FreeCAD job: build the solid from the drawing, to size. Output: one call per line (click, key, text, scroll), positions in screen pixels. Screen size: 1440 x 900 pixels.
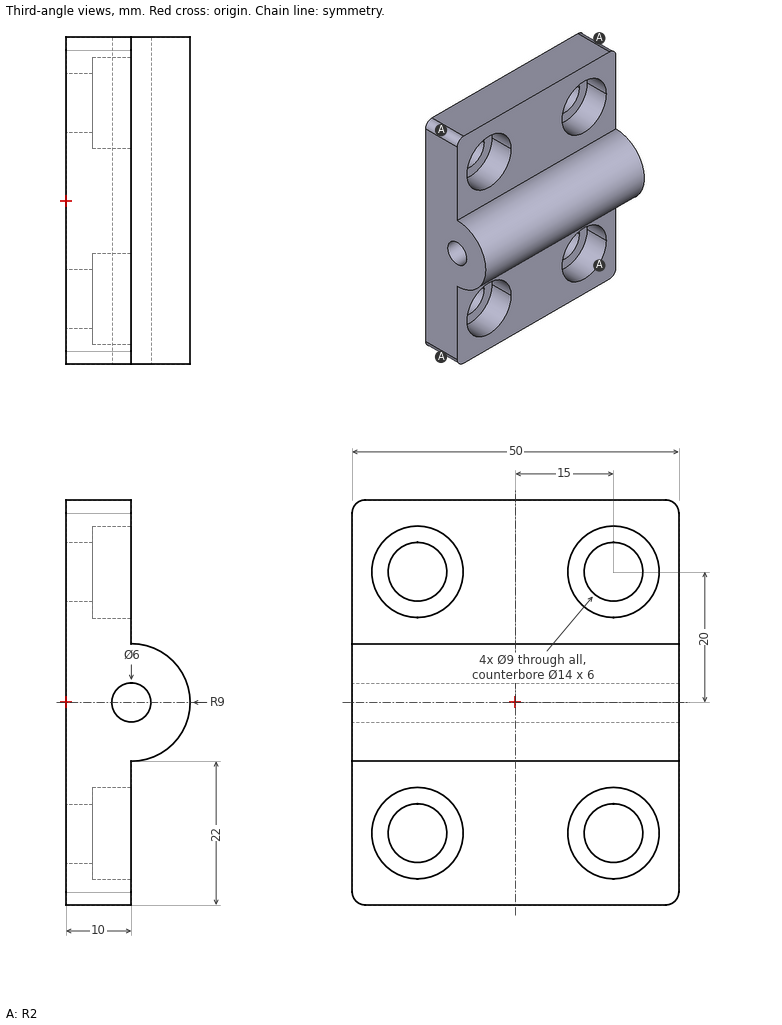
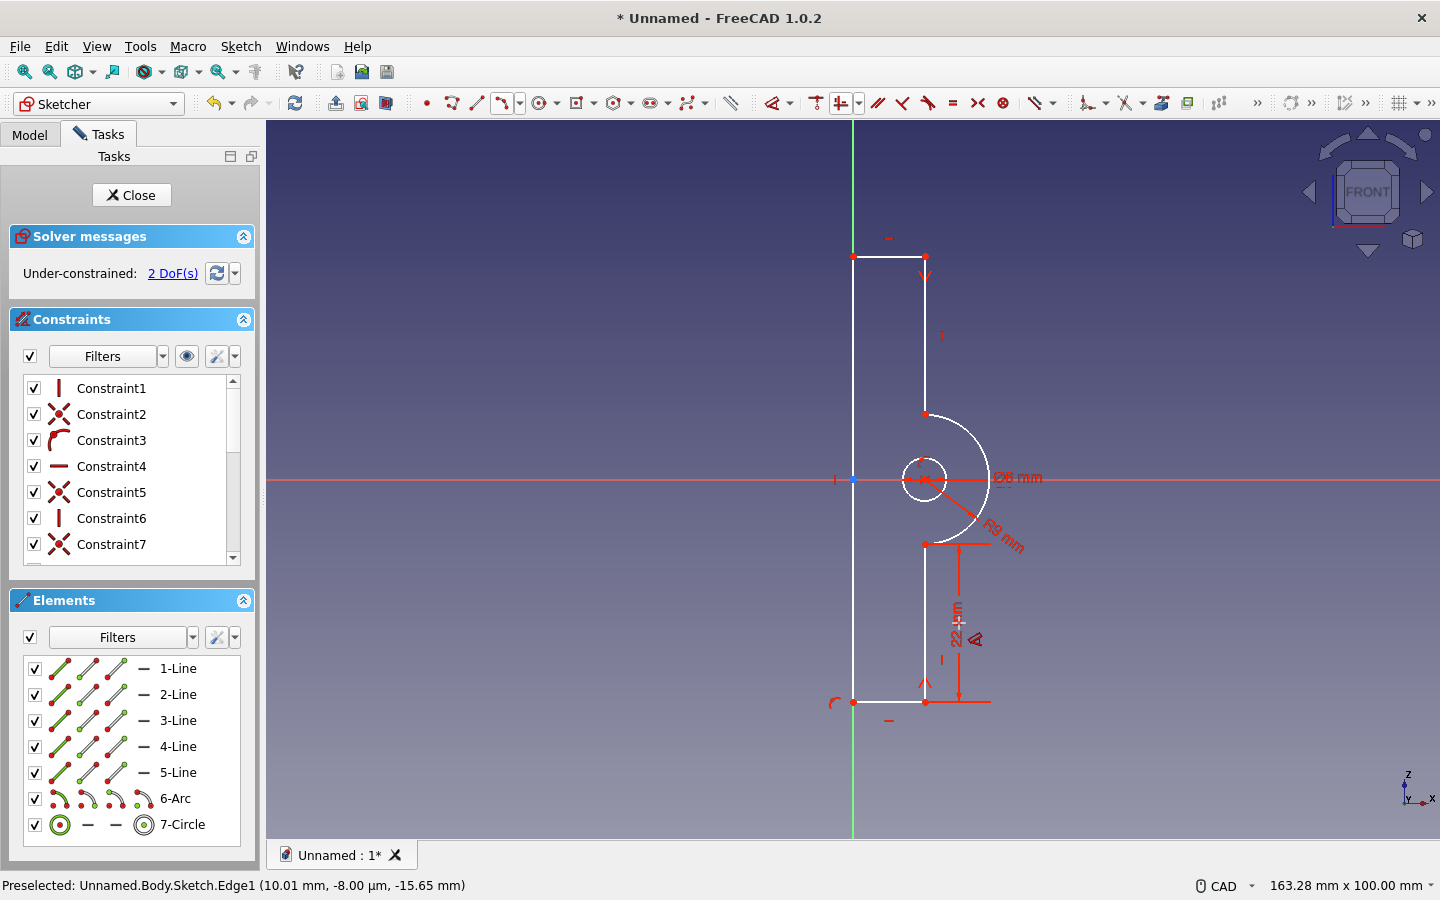
click(903, 702)
click(889, 736)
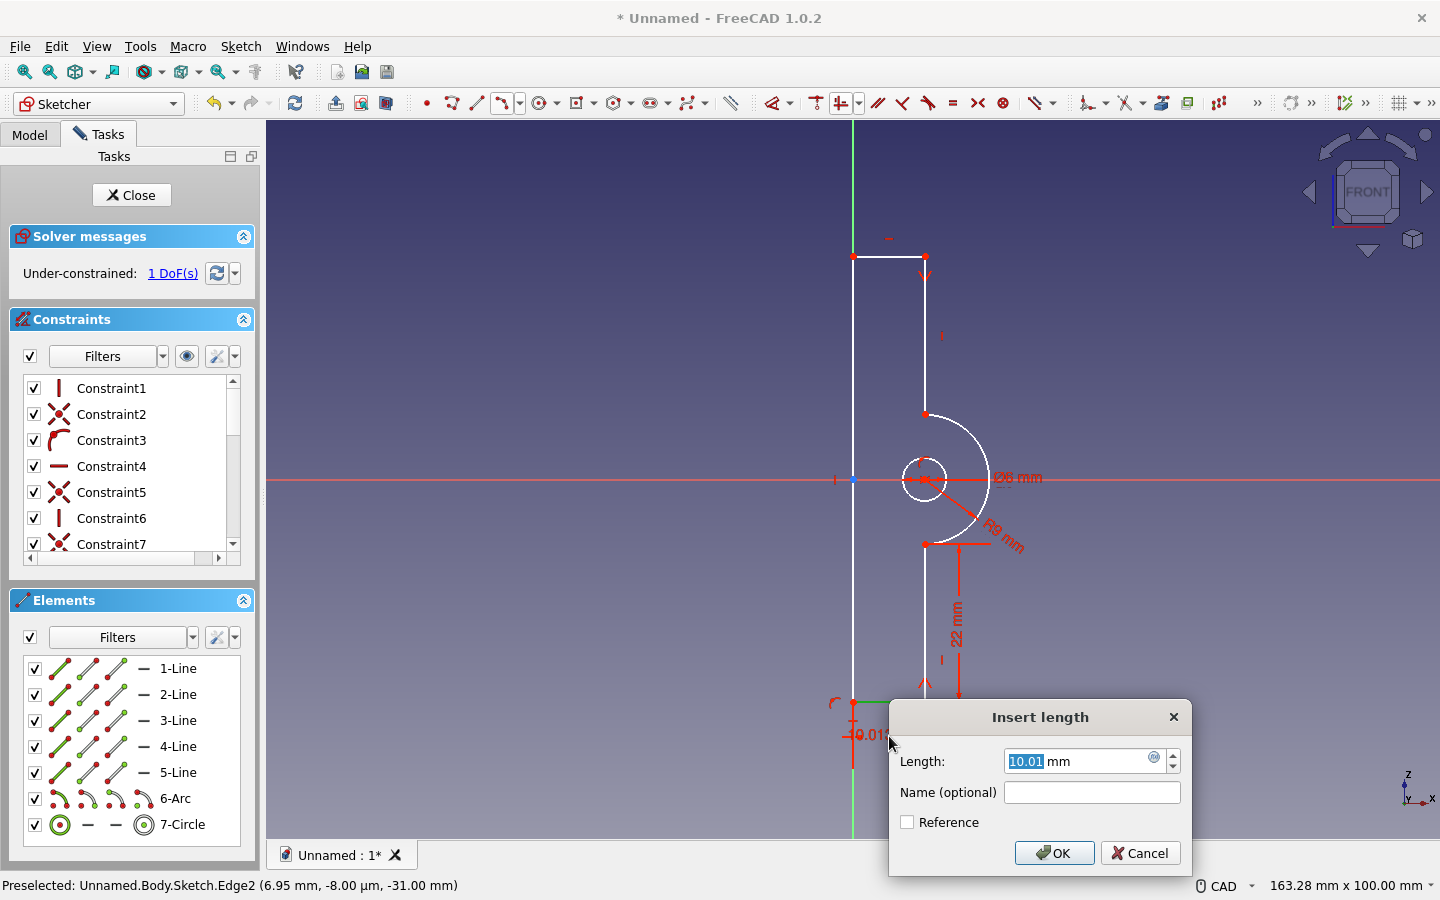
text(10)
key(Return)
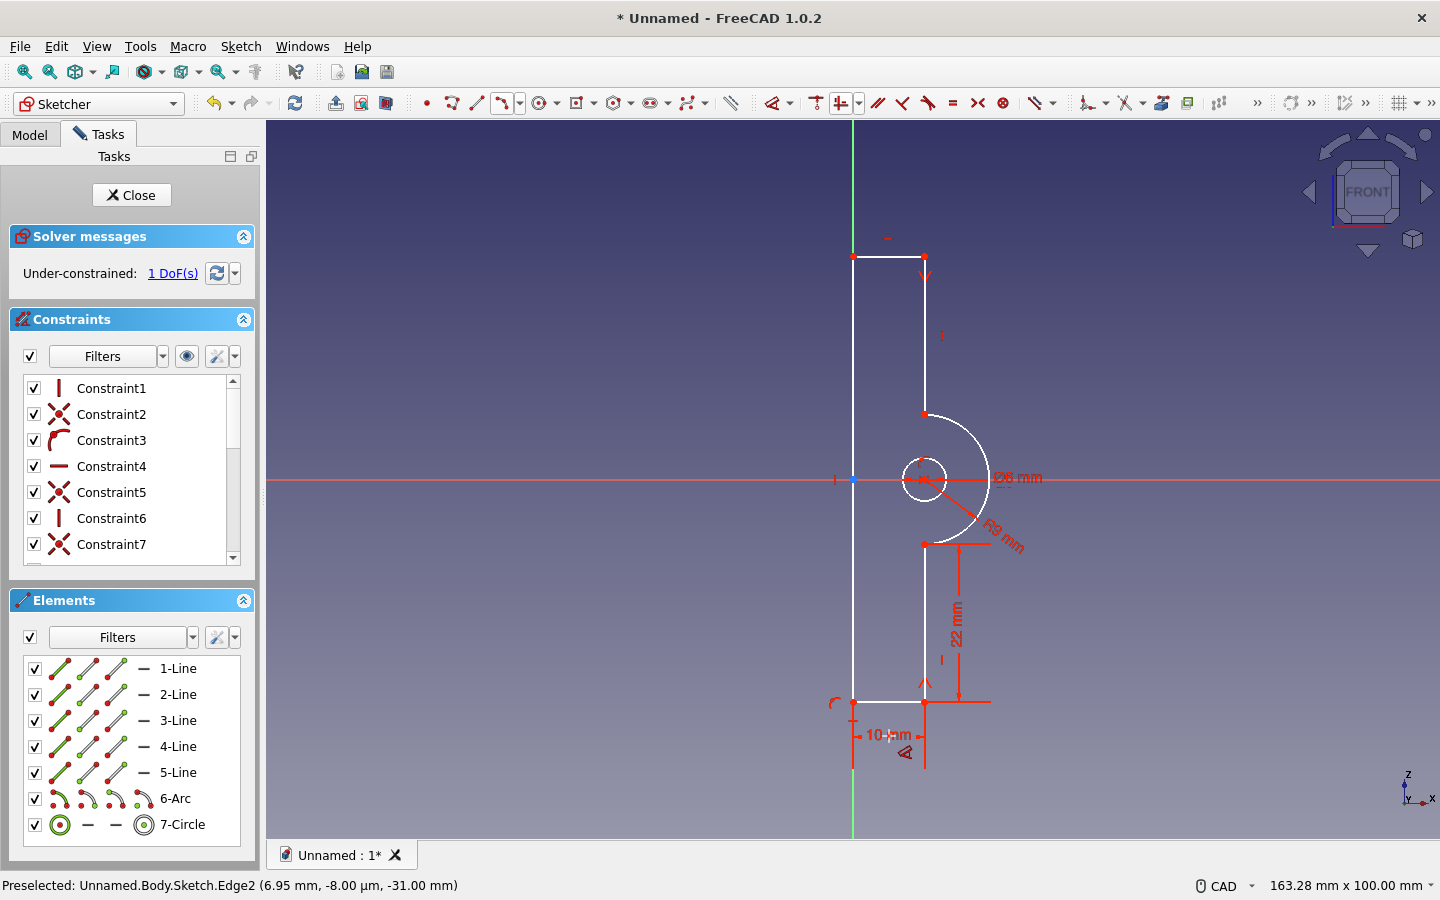
click(925, 480)
click(889, 514)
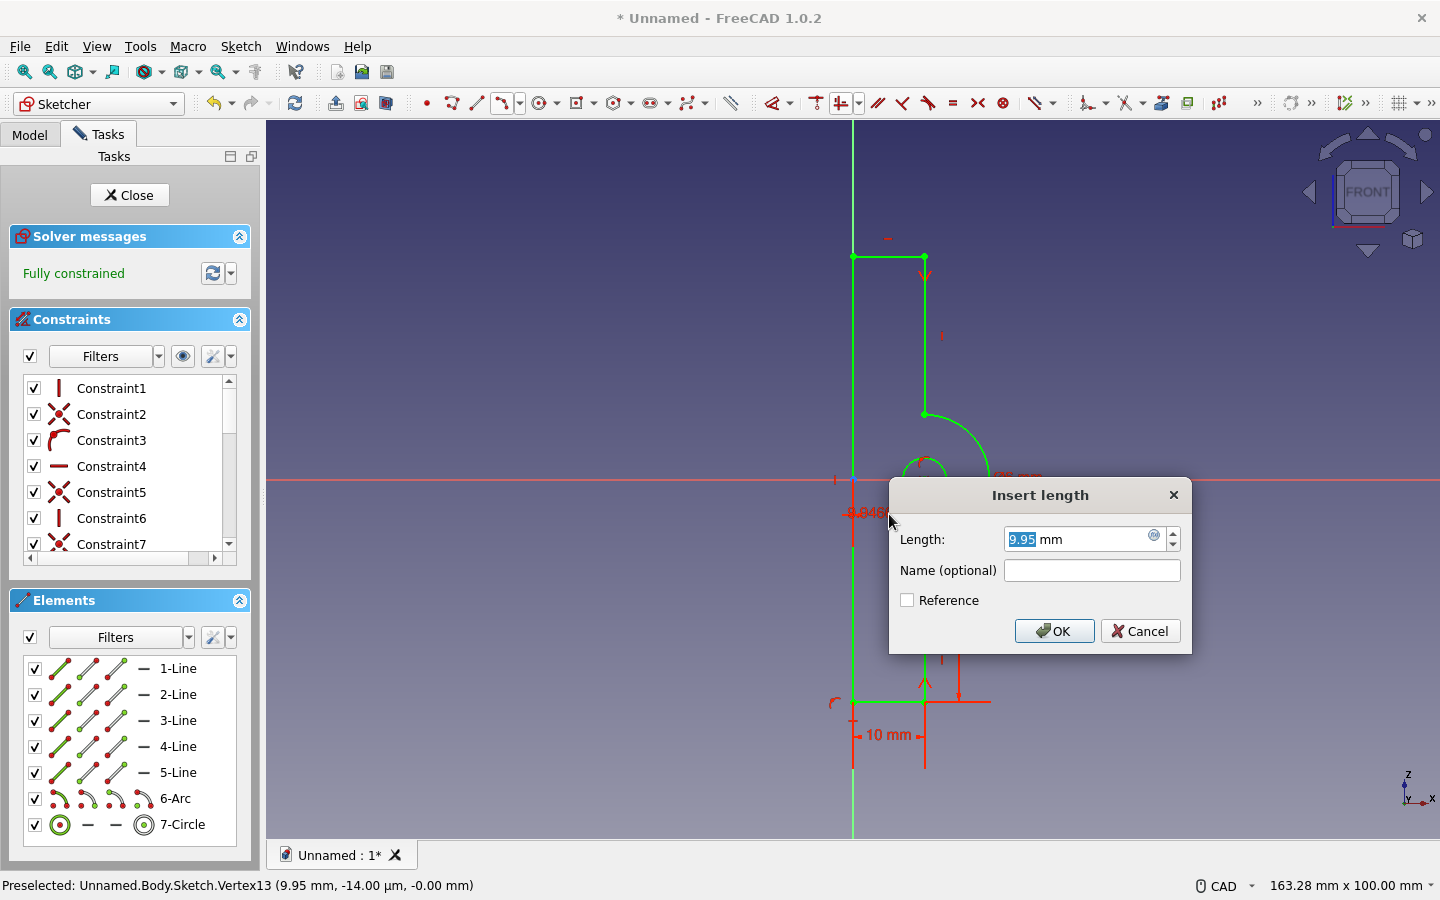
text(10)
key(Return)
key(Escape)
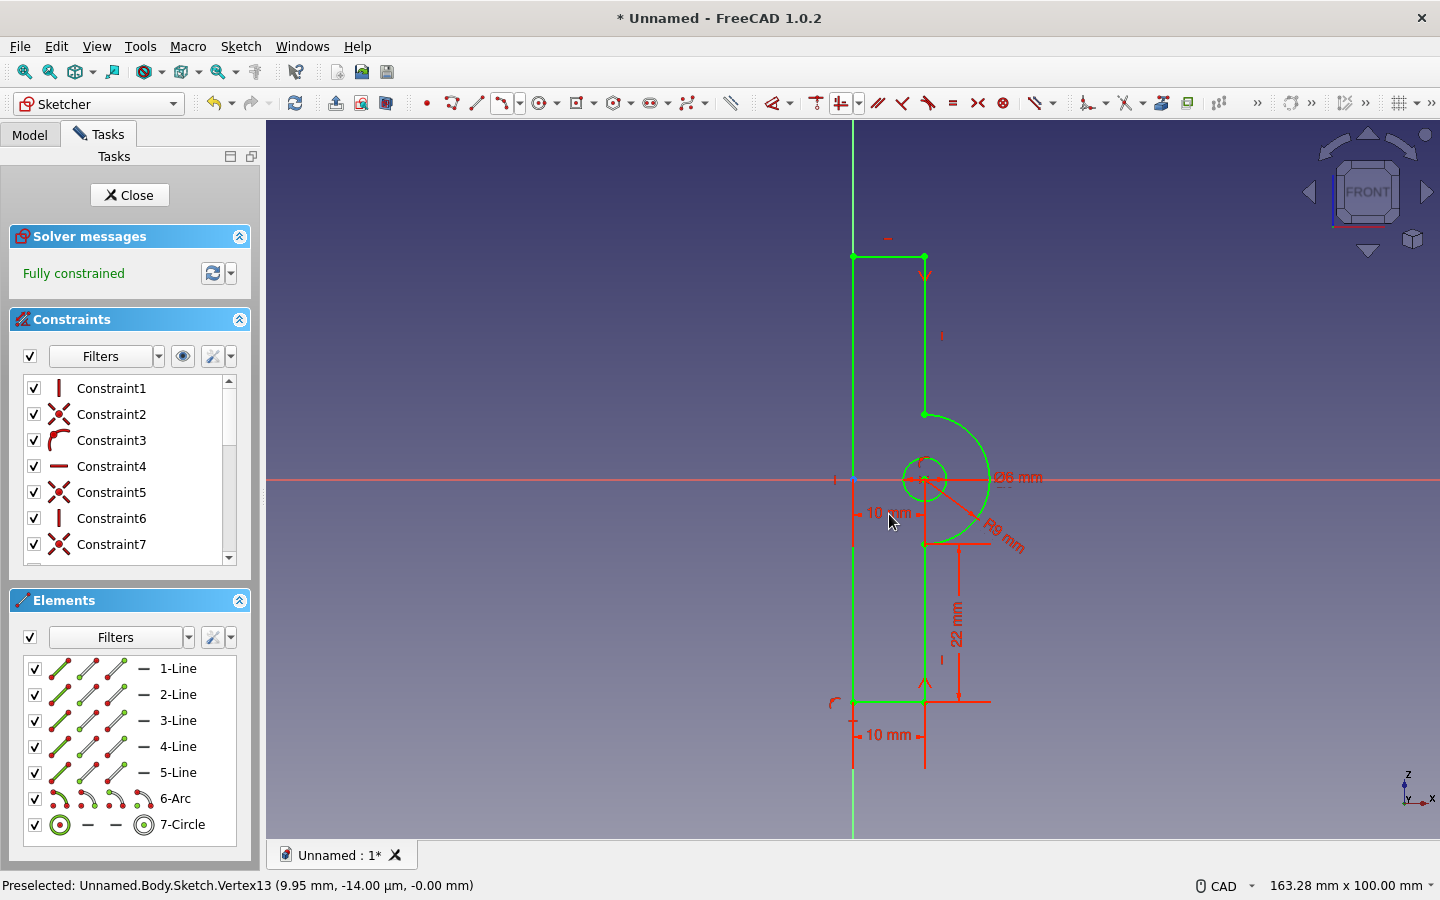
click(130, 195)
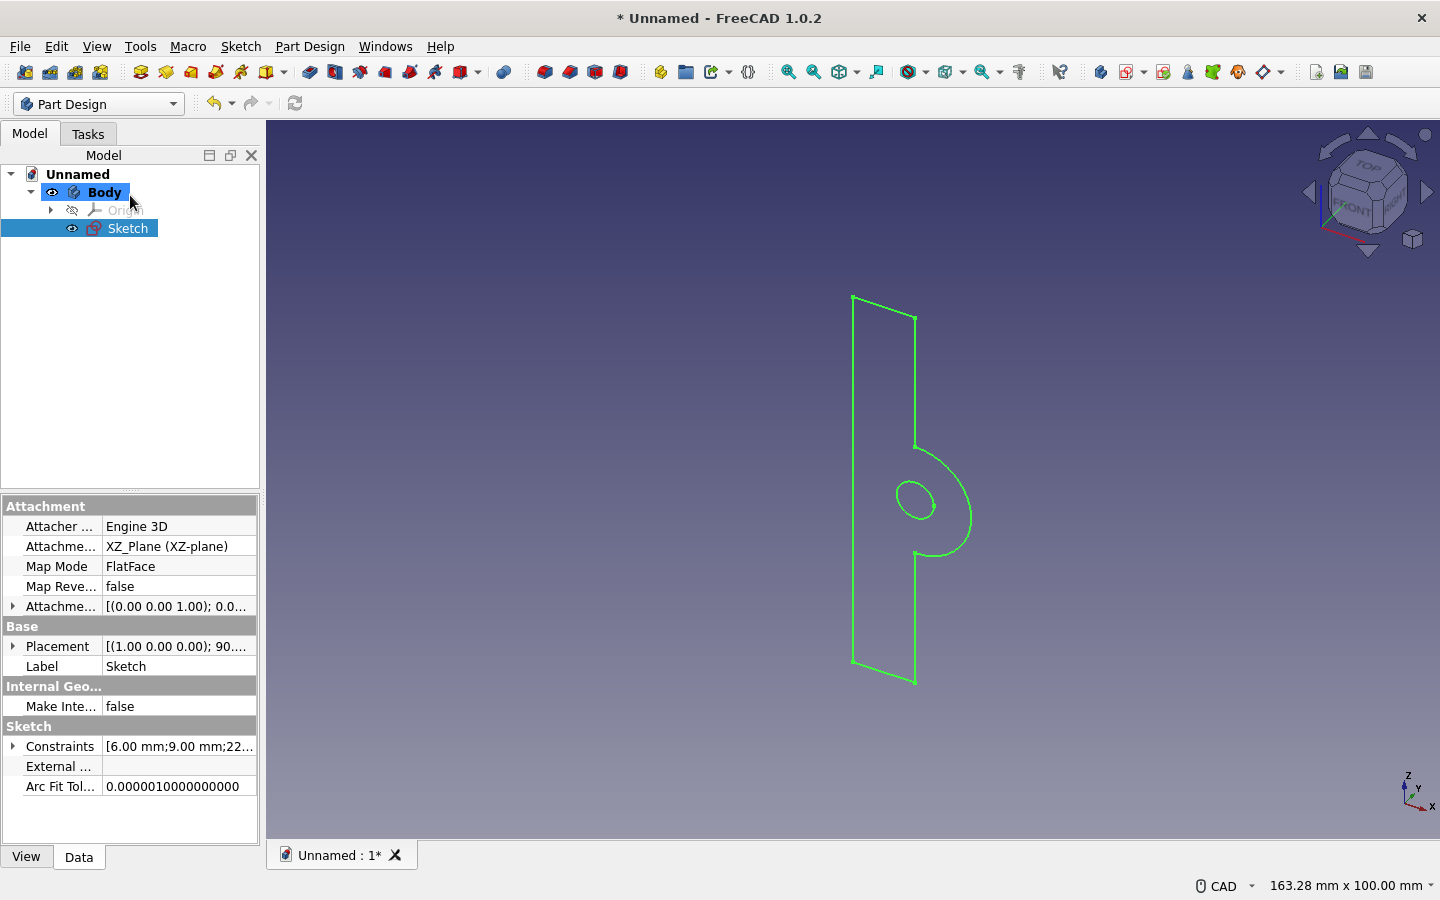
click(141, 72)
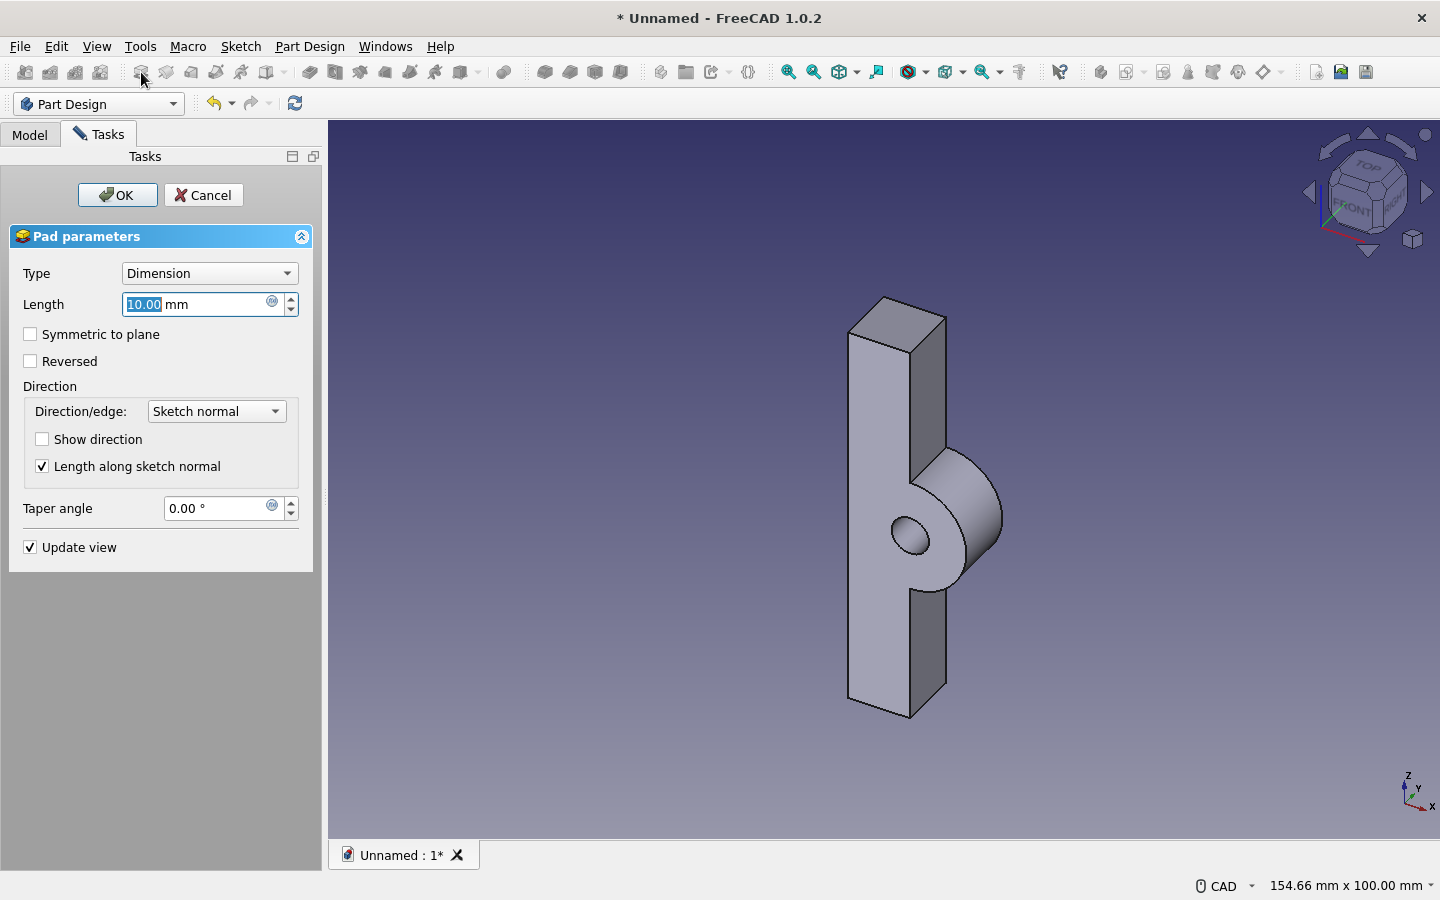
text(50)
key(Tab)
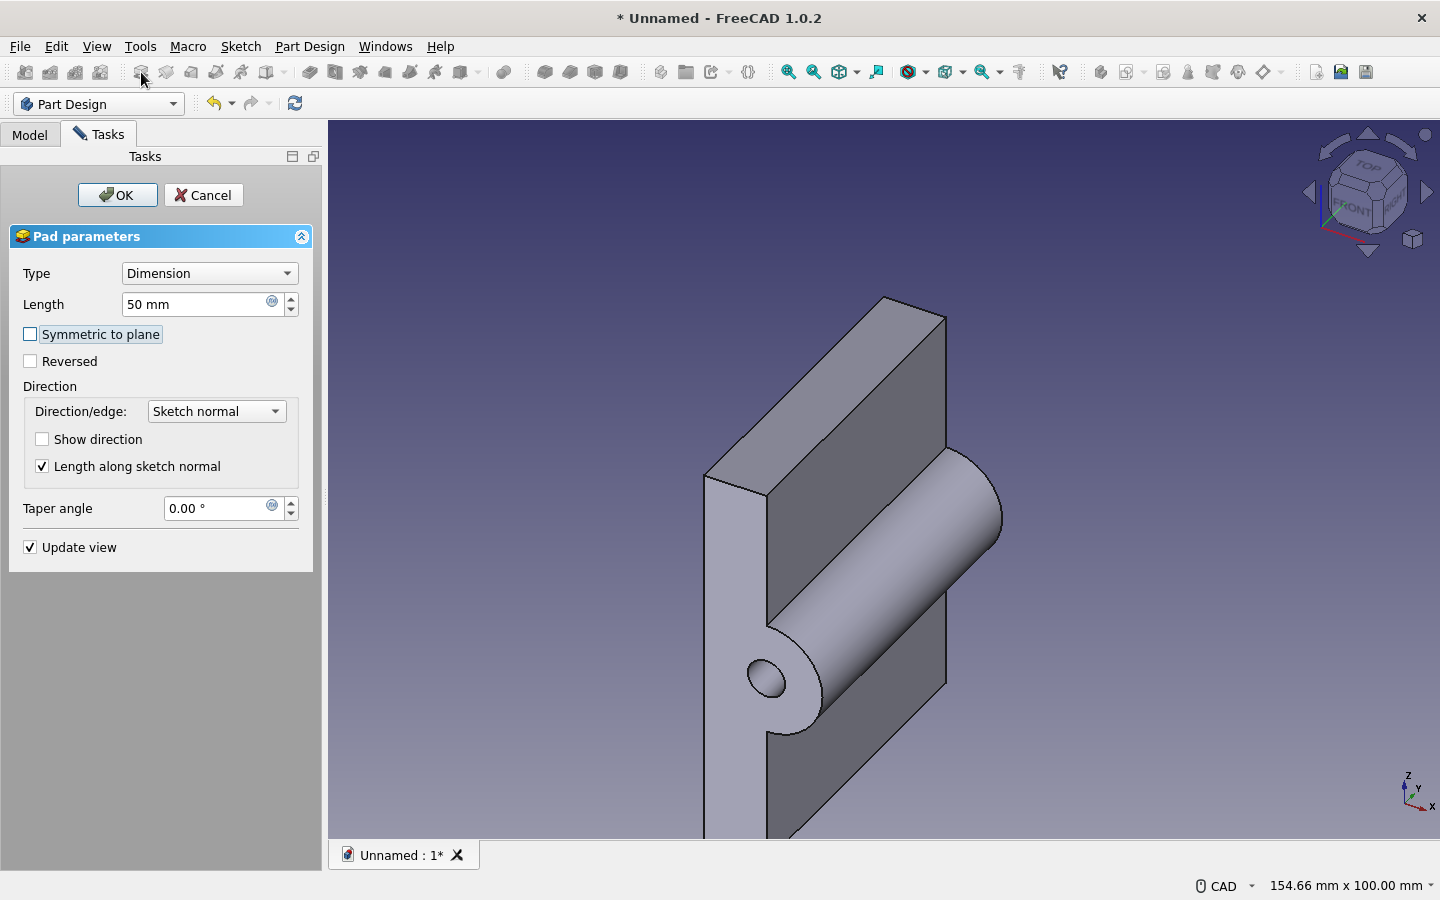
click(31, 334)